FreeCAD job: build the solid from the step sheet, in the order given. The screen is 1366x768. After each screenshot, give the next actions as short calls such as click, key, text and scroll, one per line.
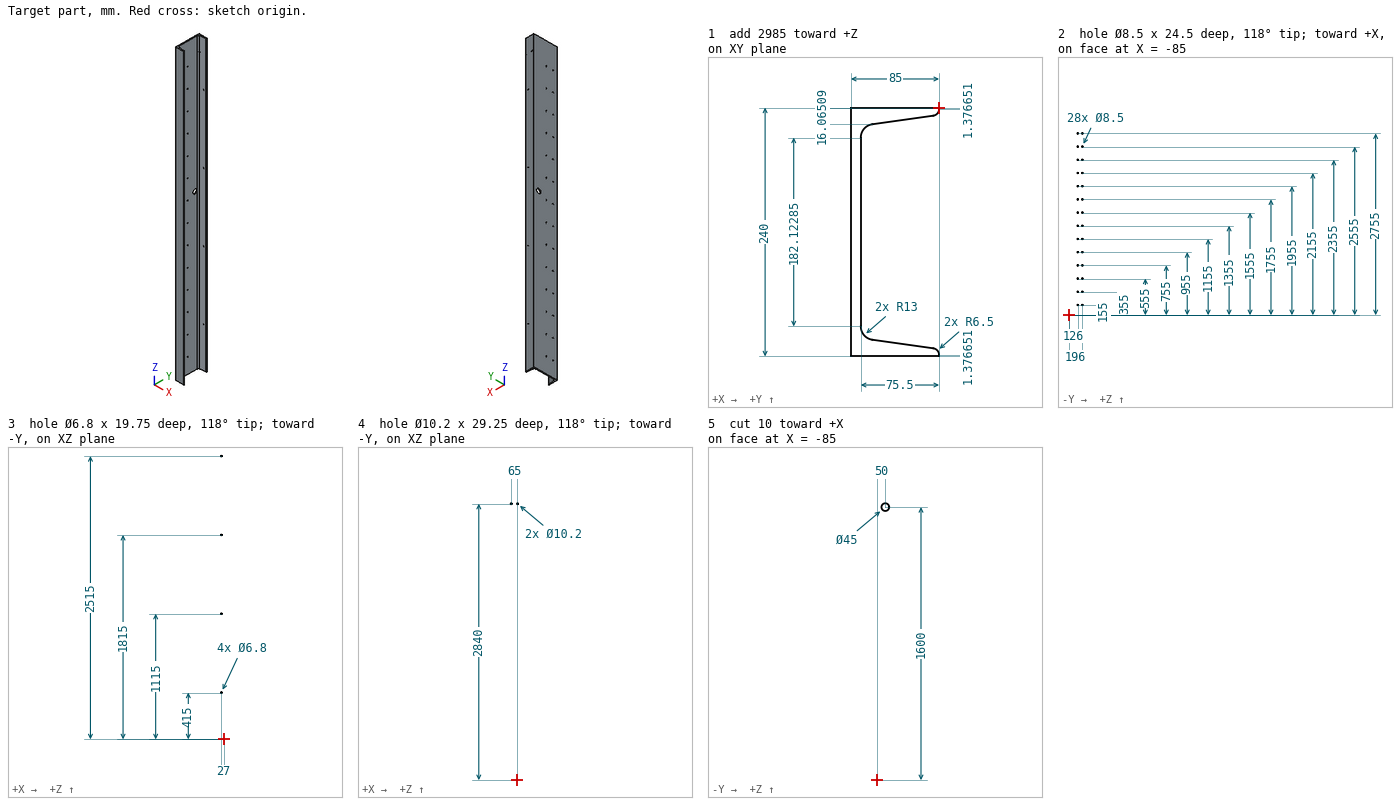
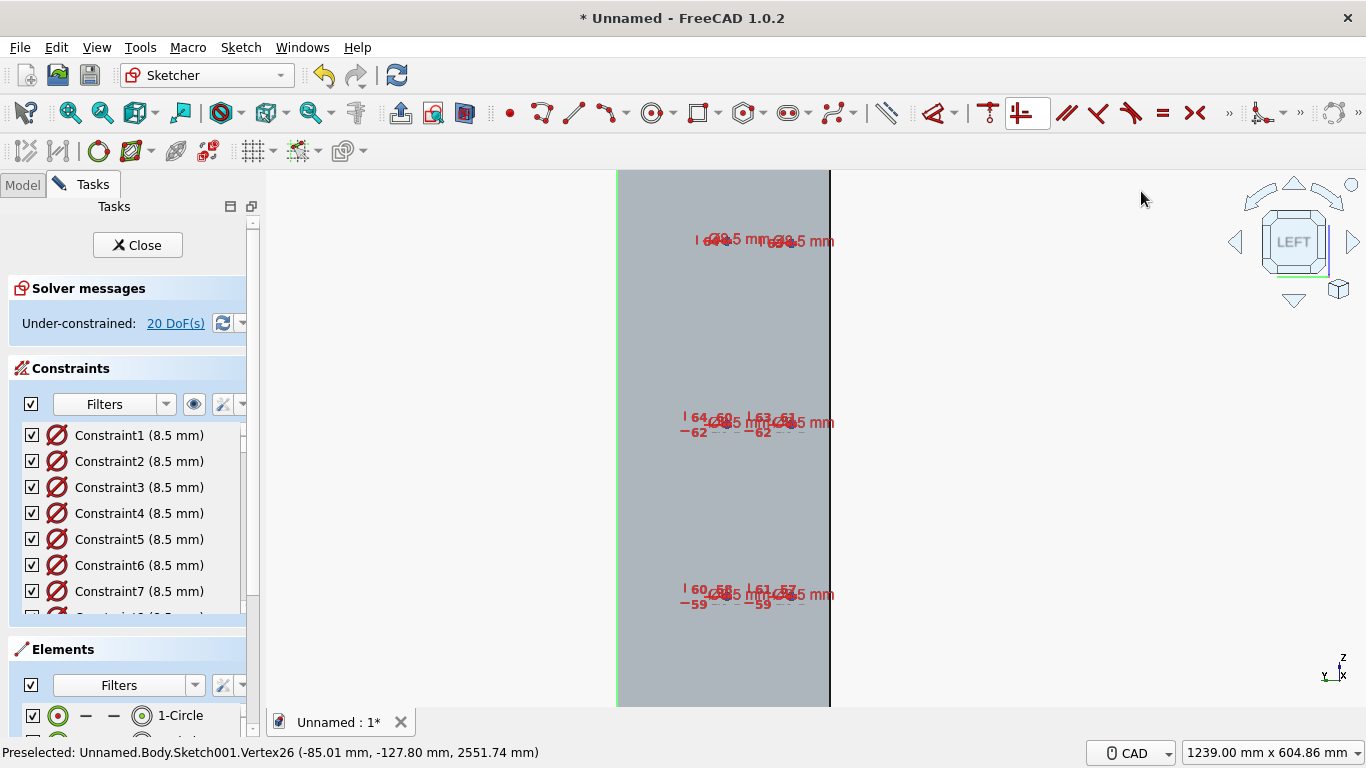
scroll(754, 307, down, 10)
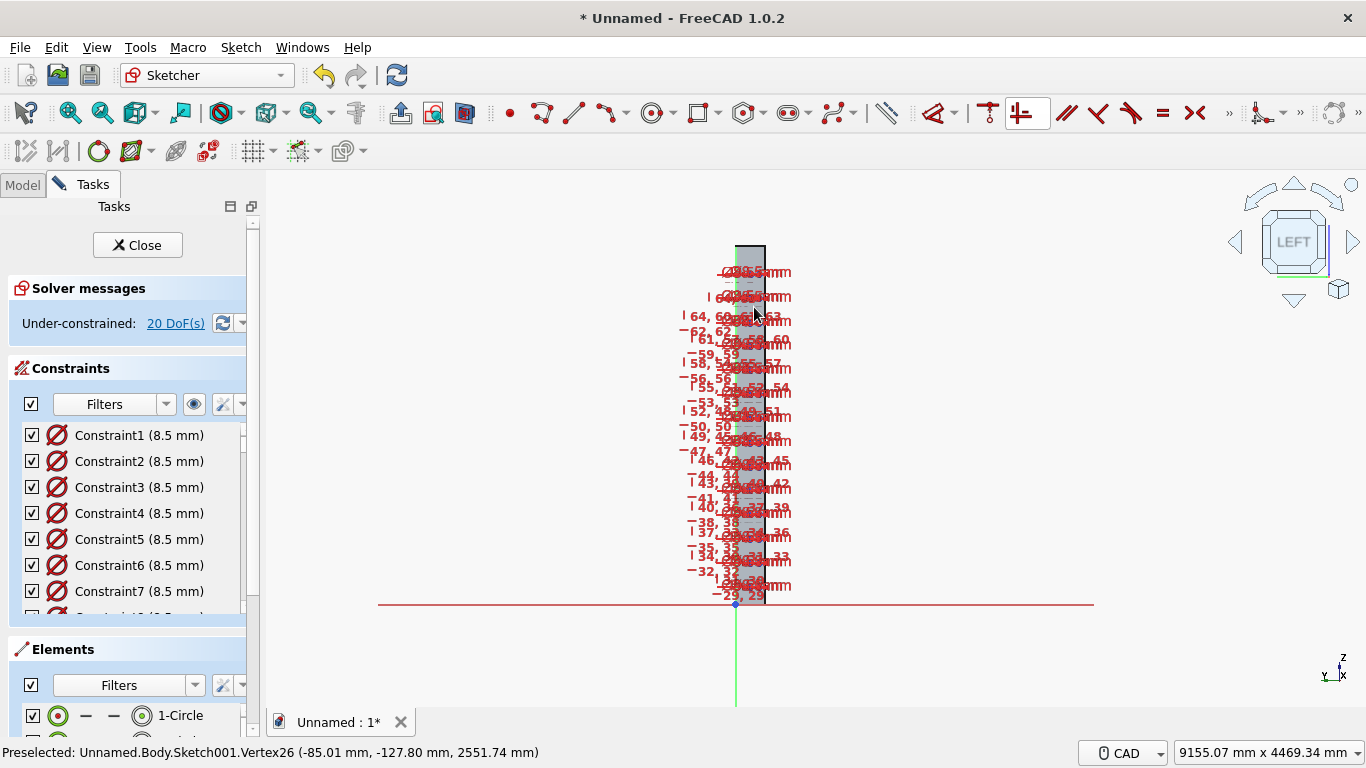
scroll(759, 299, up, 2)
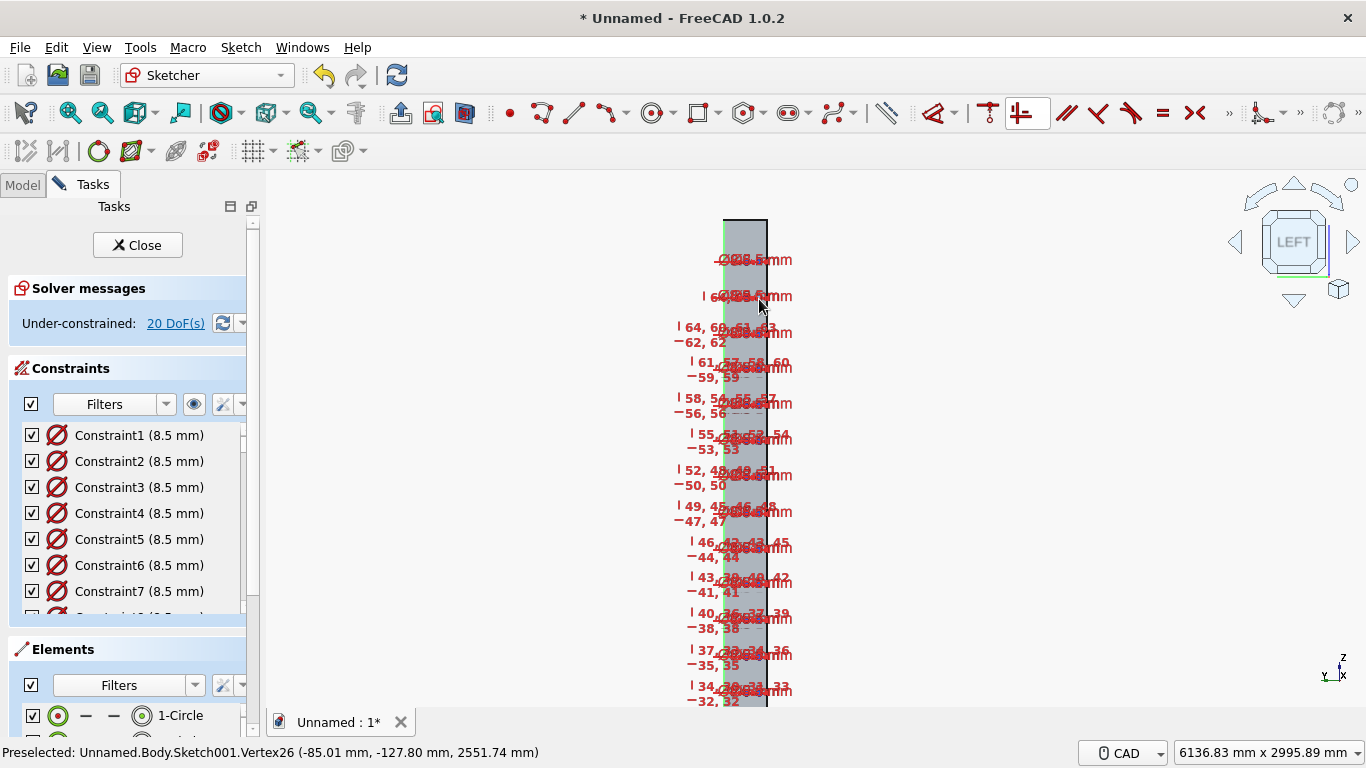
click(759, 298)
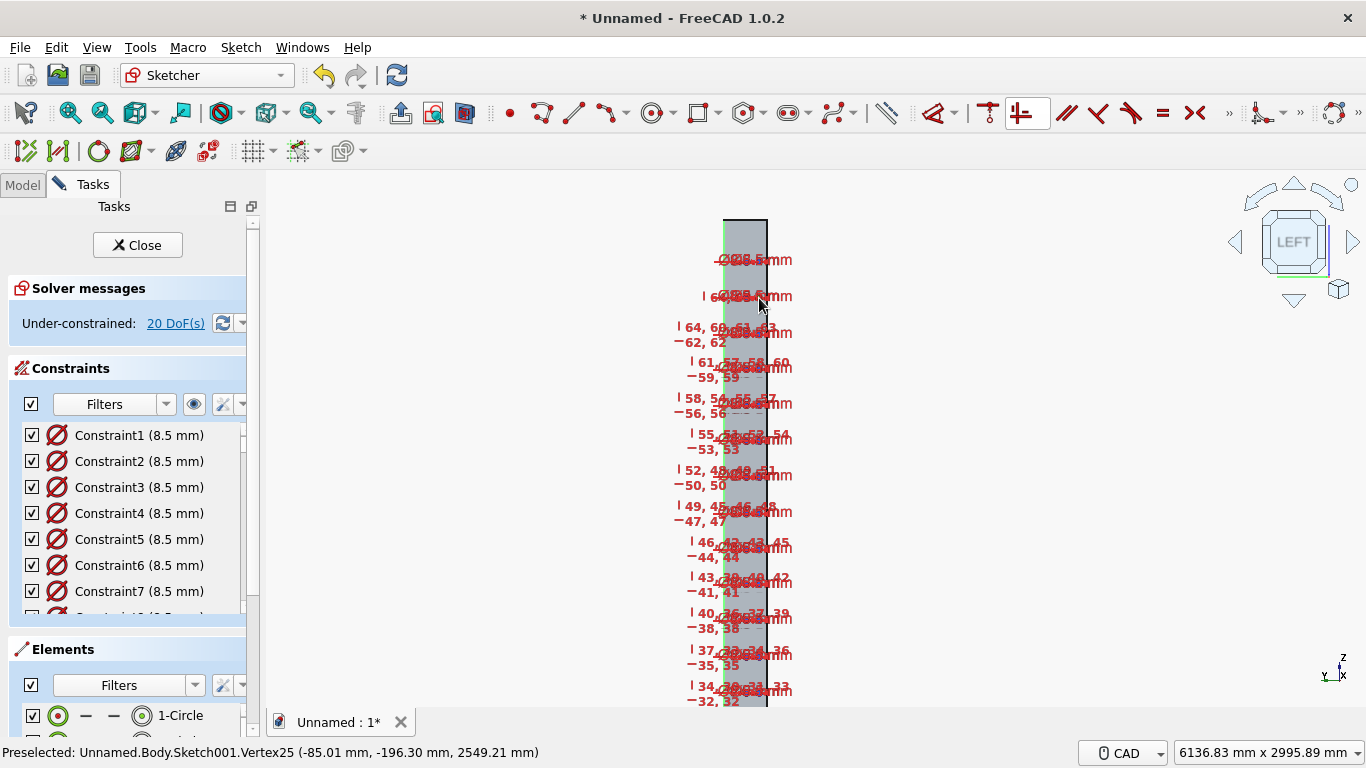
scroll(746, 298, up, 4)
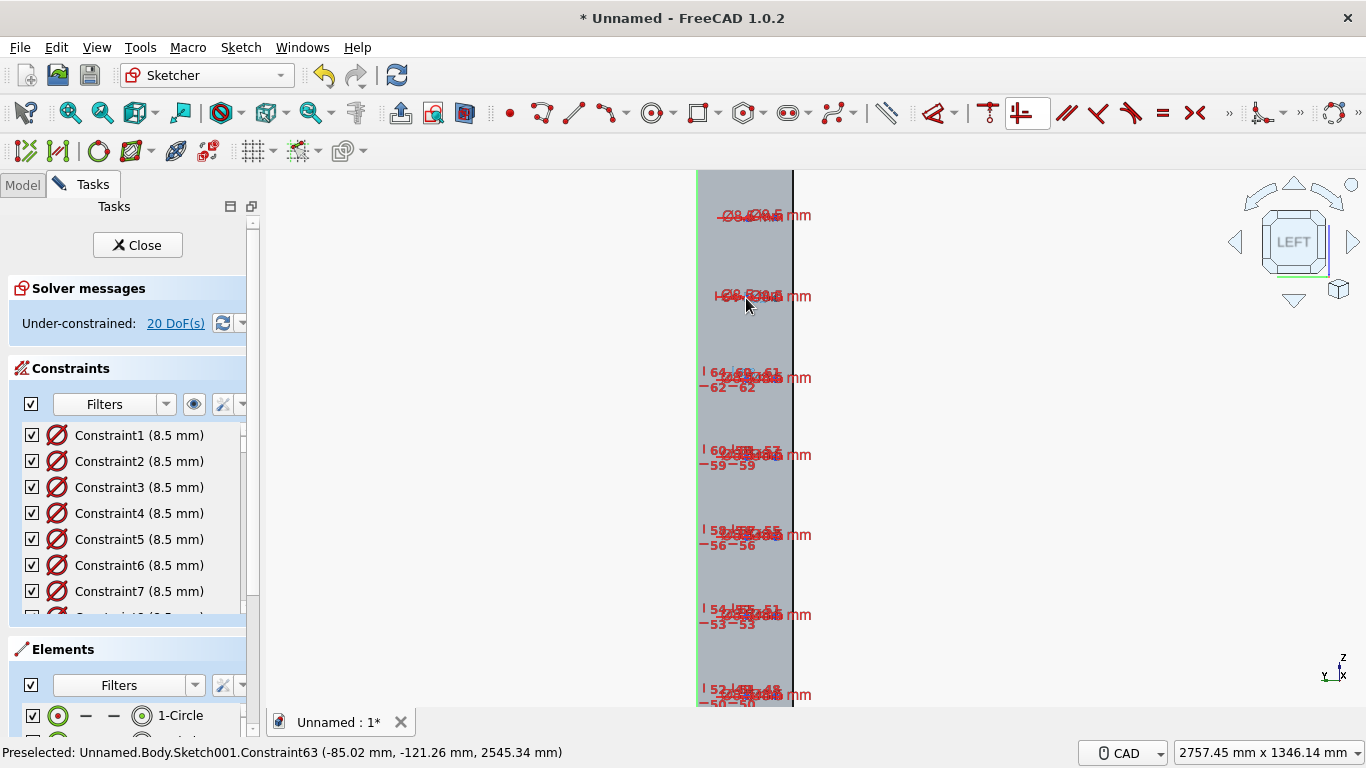
scroll(746, 297, up, 4)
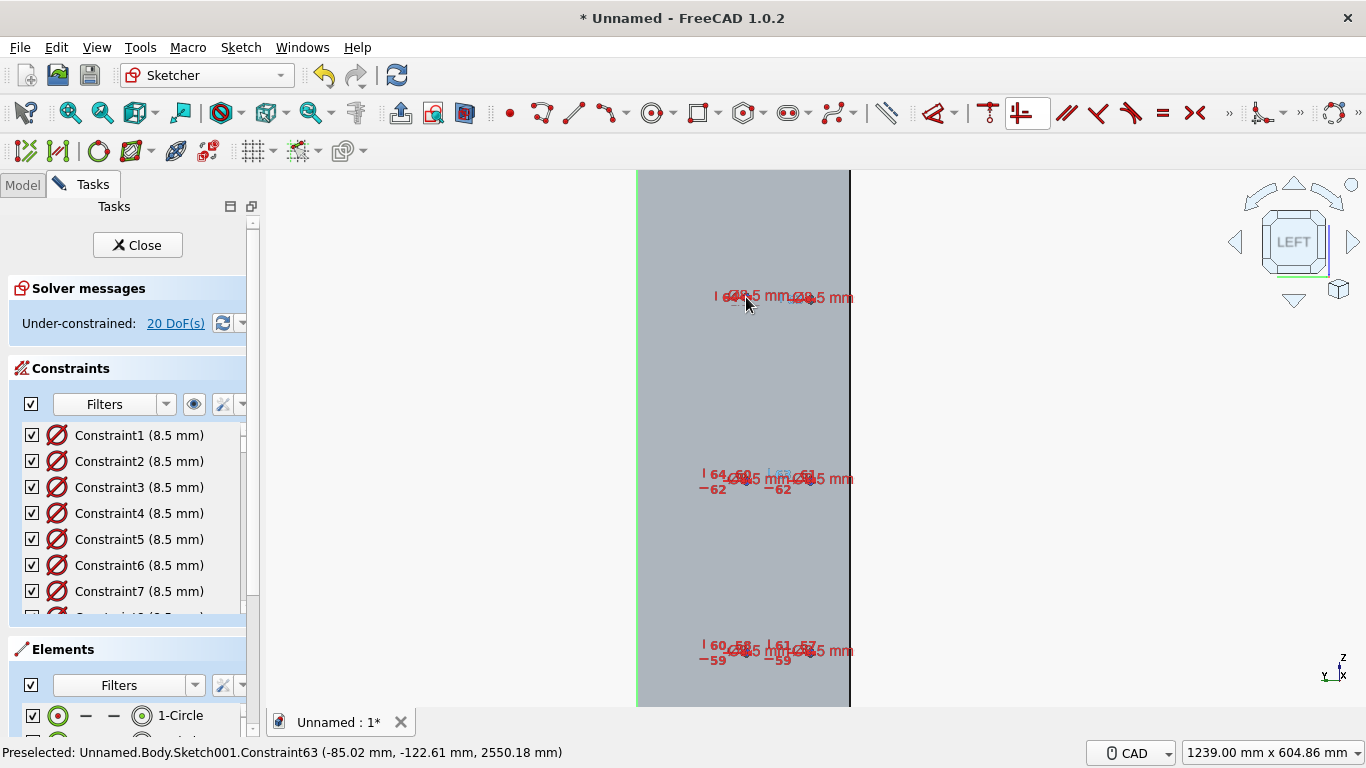
click(746, 298)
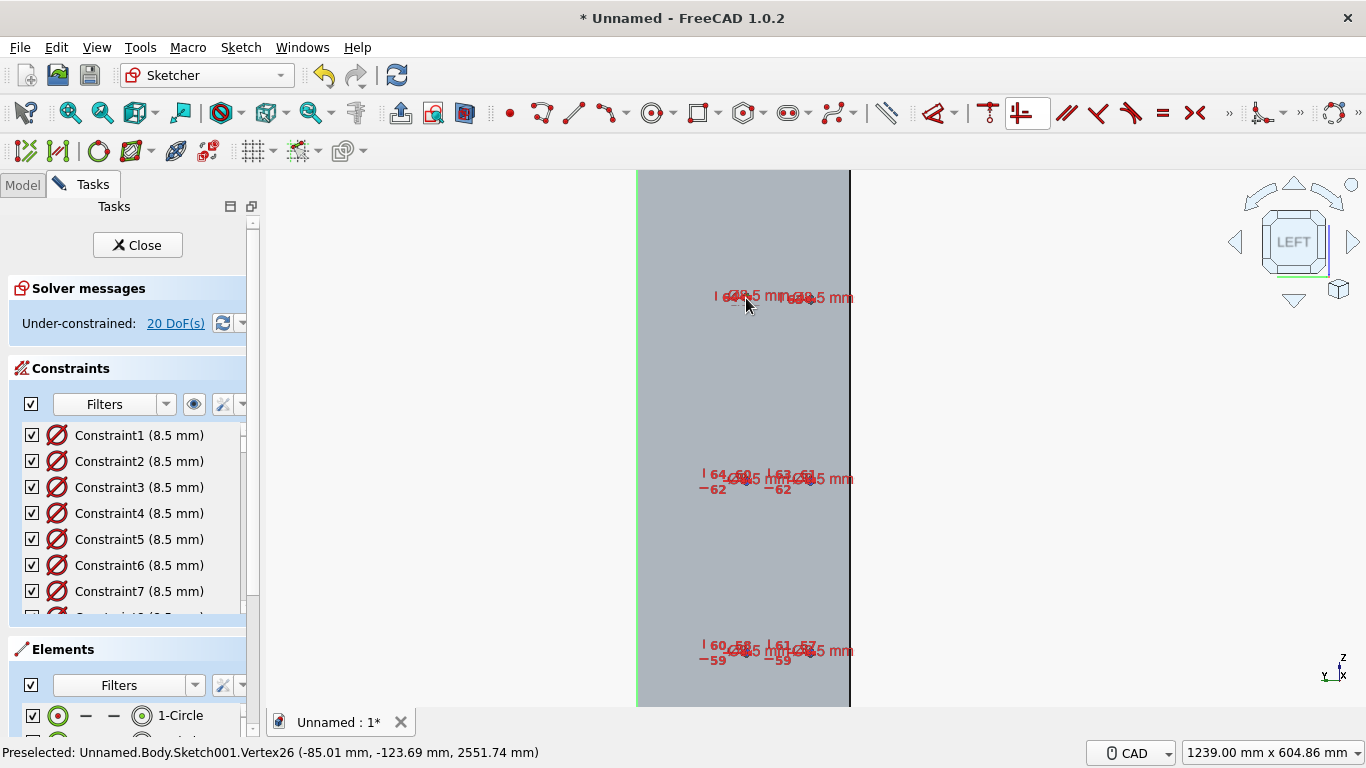
click(1044, 114)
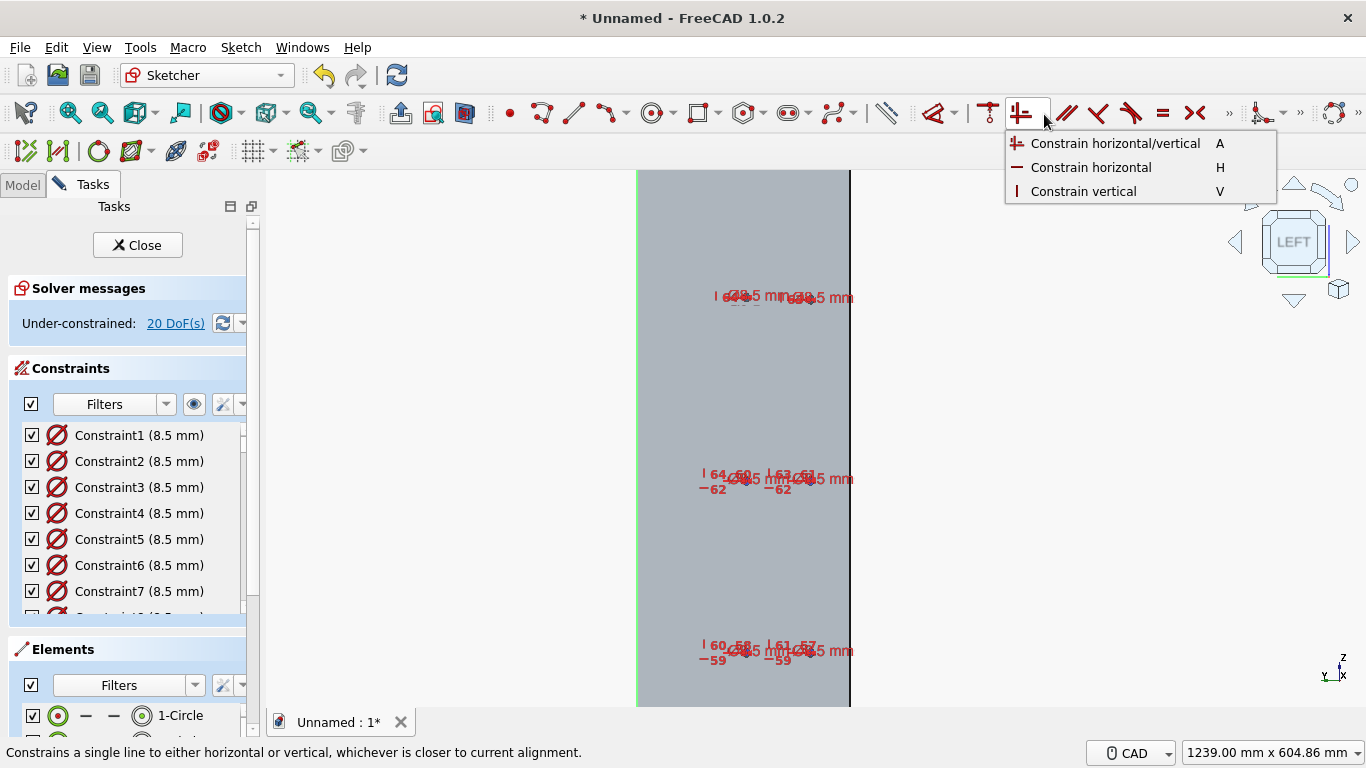
click(1141, 167)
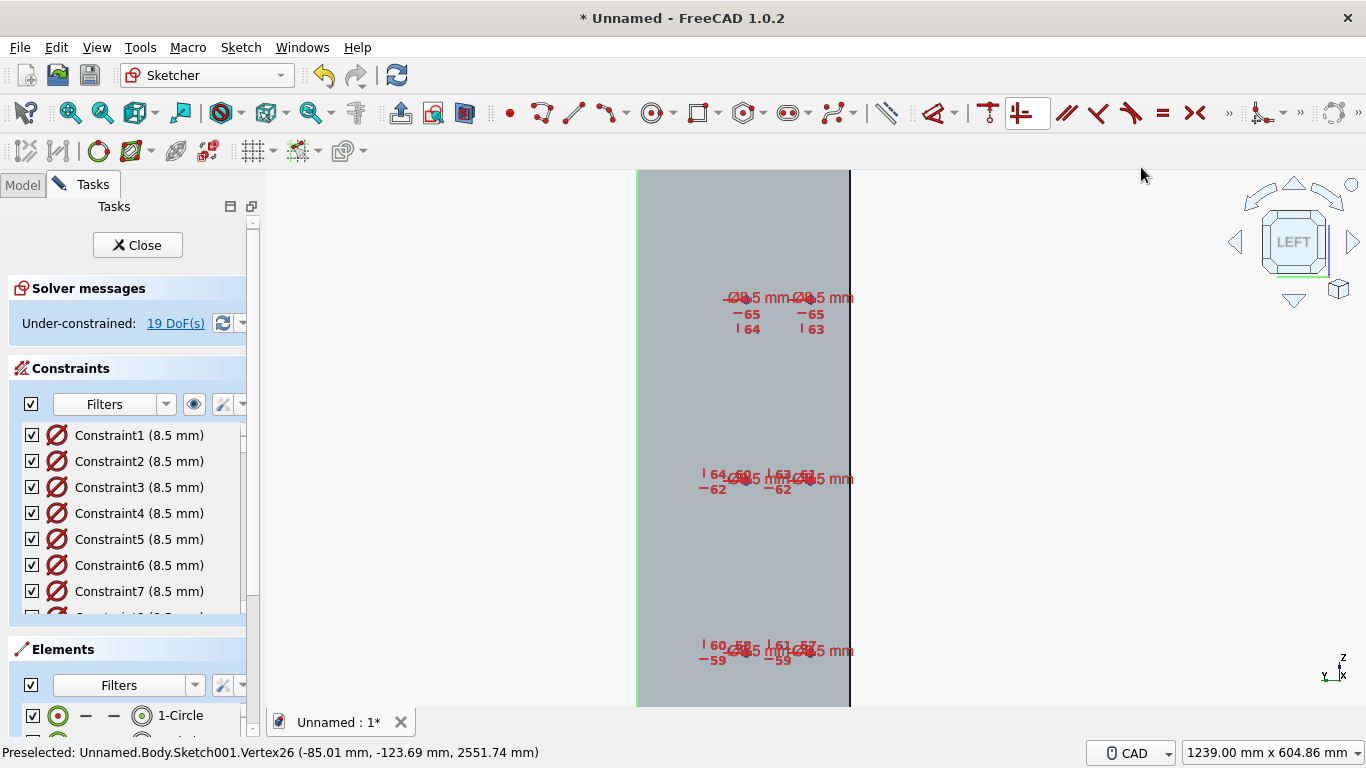
scroll(751, 298, down, 10)